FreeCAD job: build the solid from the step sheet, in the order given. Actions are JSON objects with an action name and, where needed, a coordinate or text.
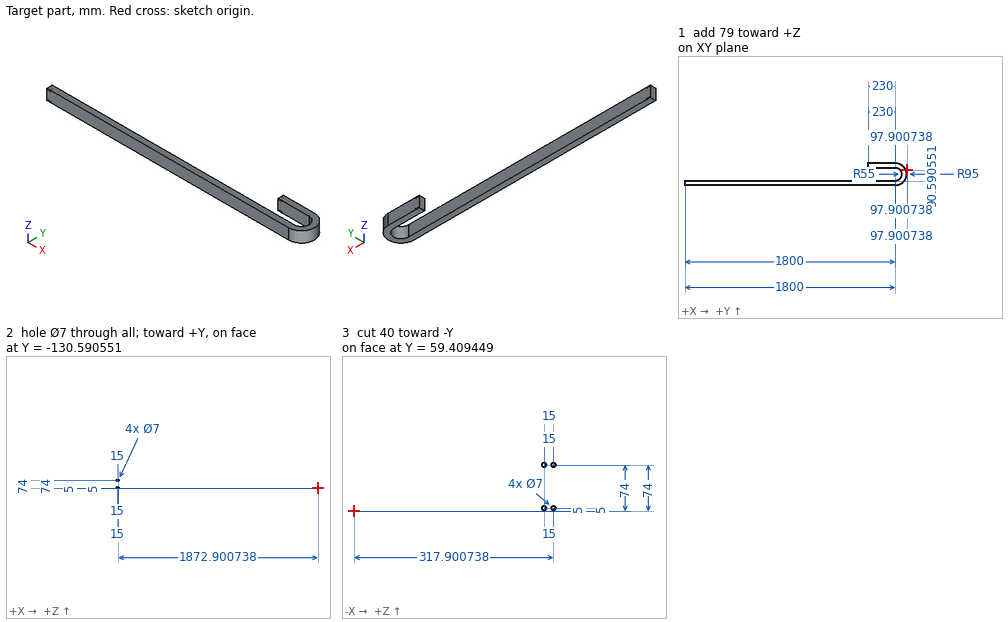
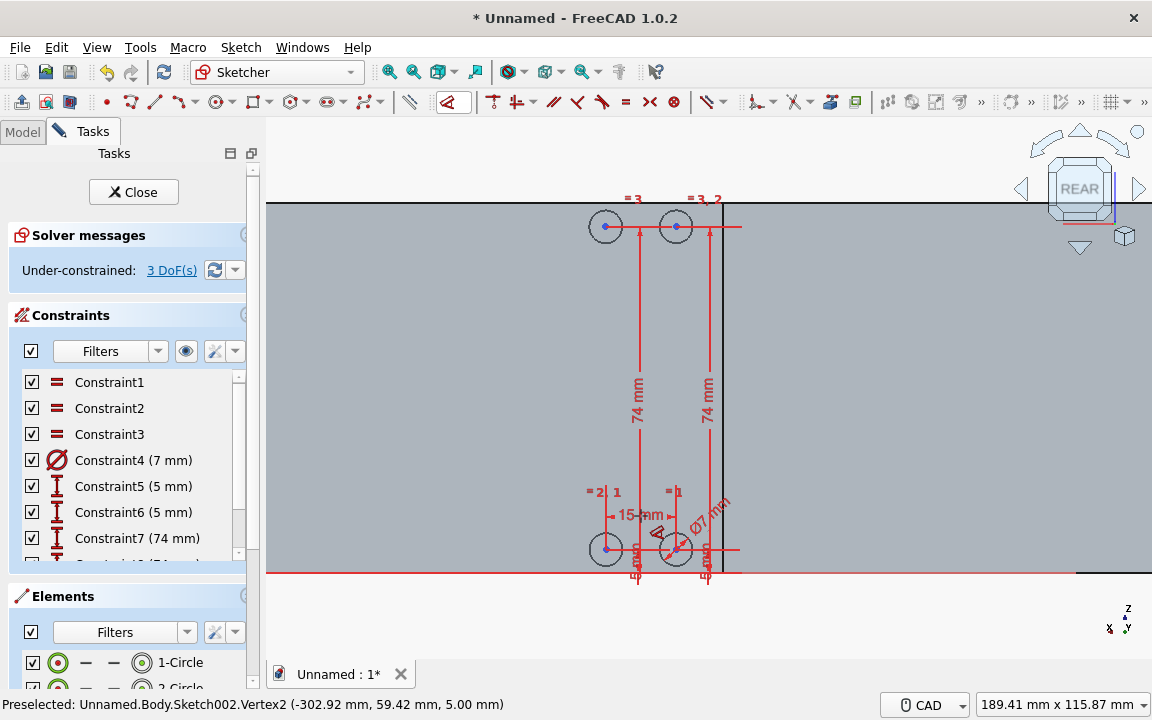
{"action": "left_click", "coordinate": [606, 550]}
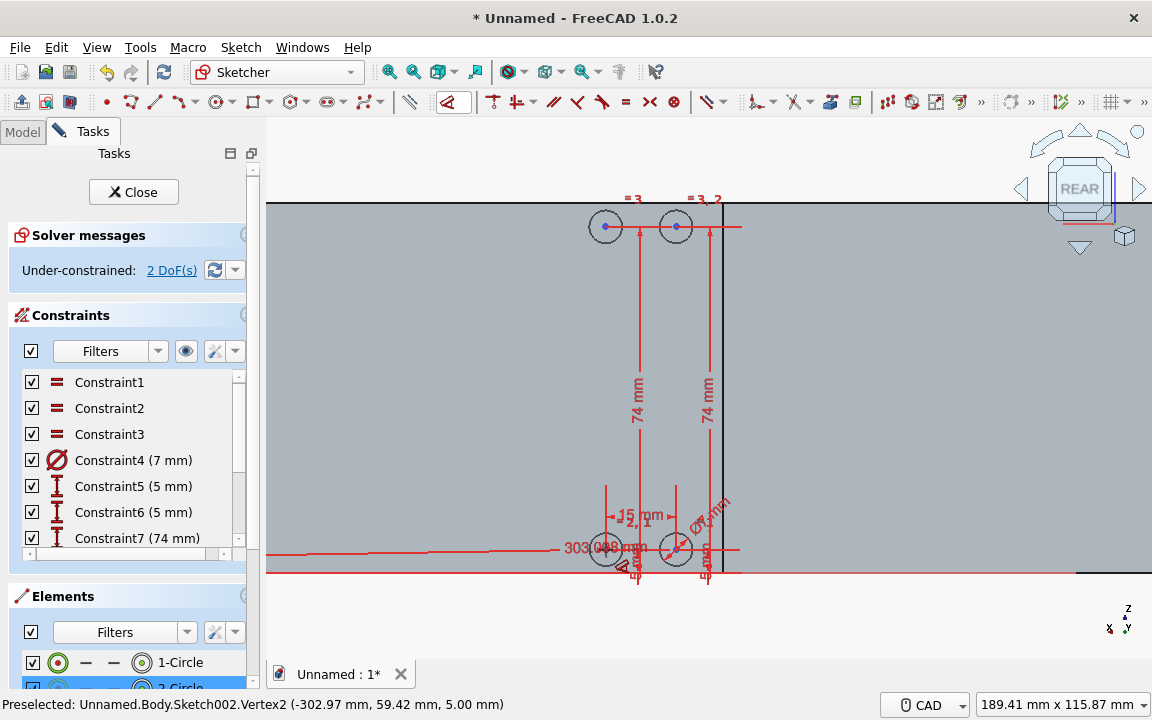
{"action": "left_click", "coordinate": [676, 227]}
{"action": "left_click", "coordinate": [641, 193]}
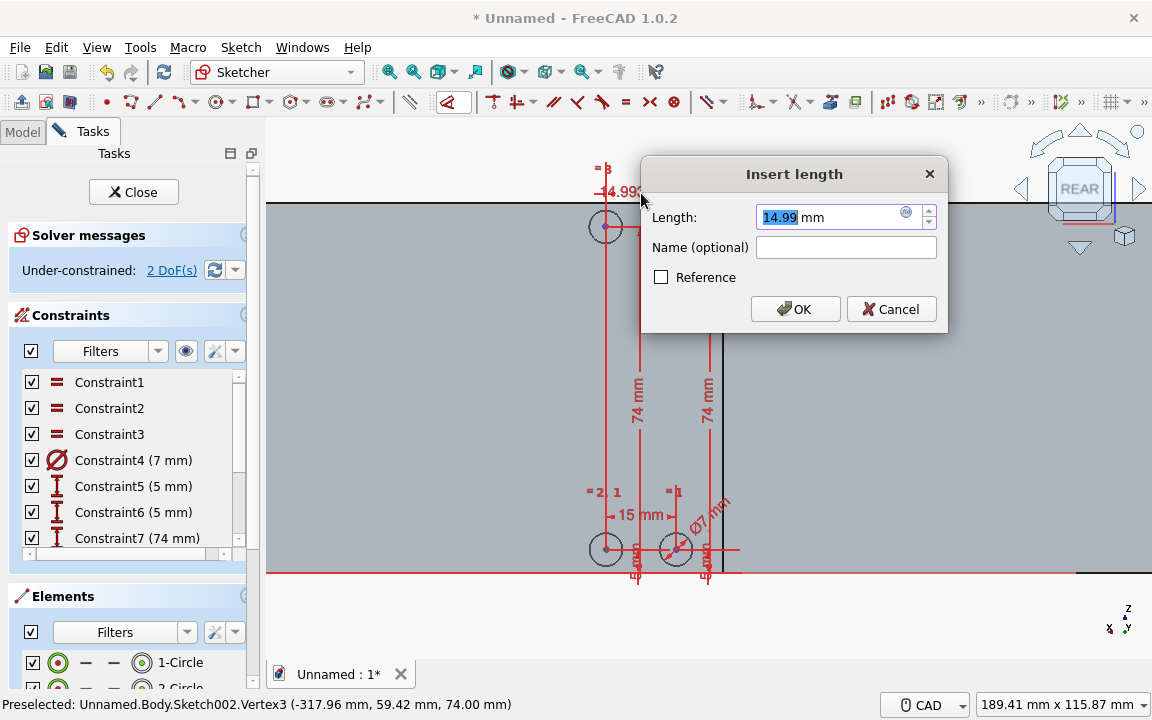
{"action": "type", "text": "15"}
{"action": "key", "text": "Return"}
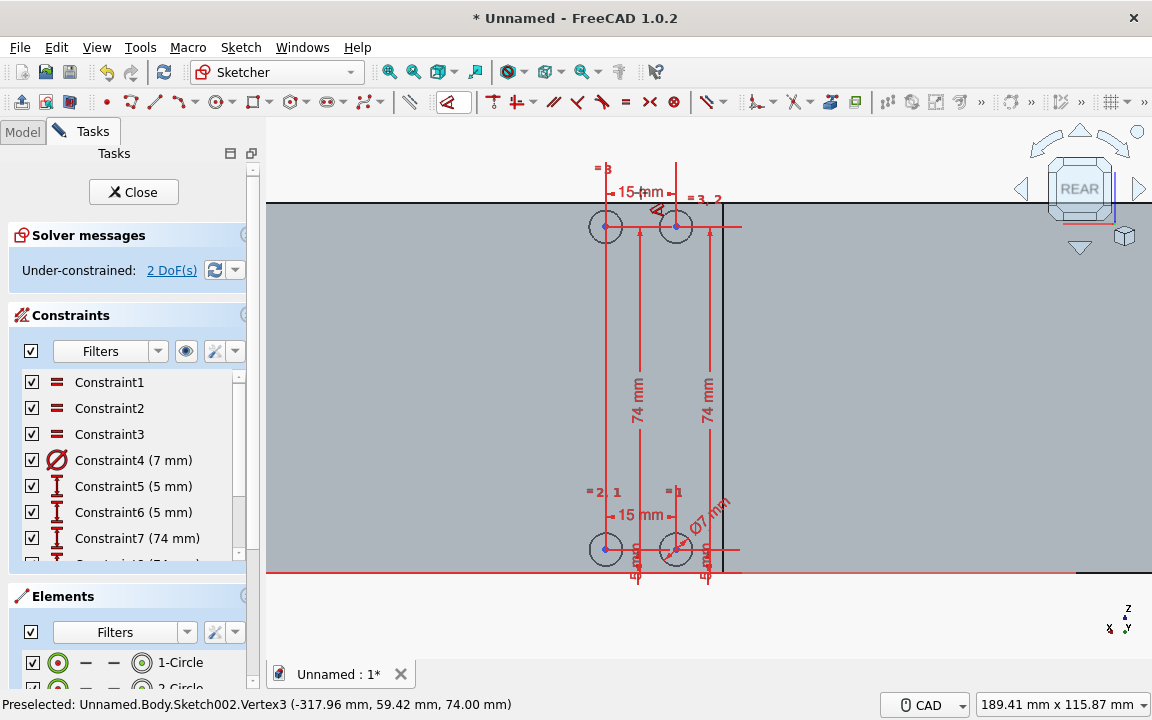
{"action": "left_click", "coordinate": [676, 227]}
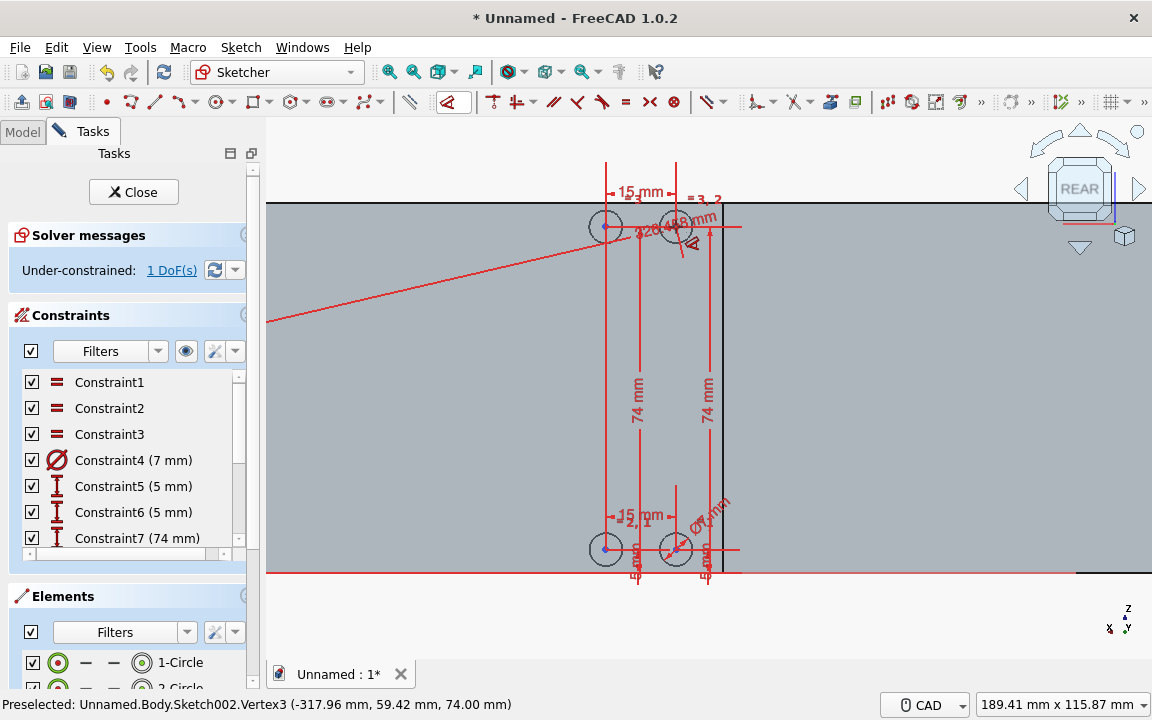
{"action": "left_click", "coordinate": [606, 227]}
{"action": "left_click", "coordinate": [641, 261]}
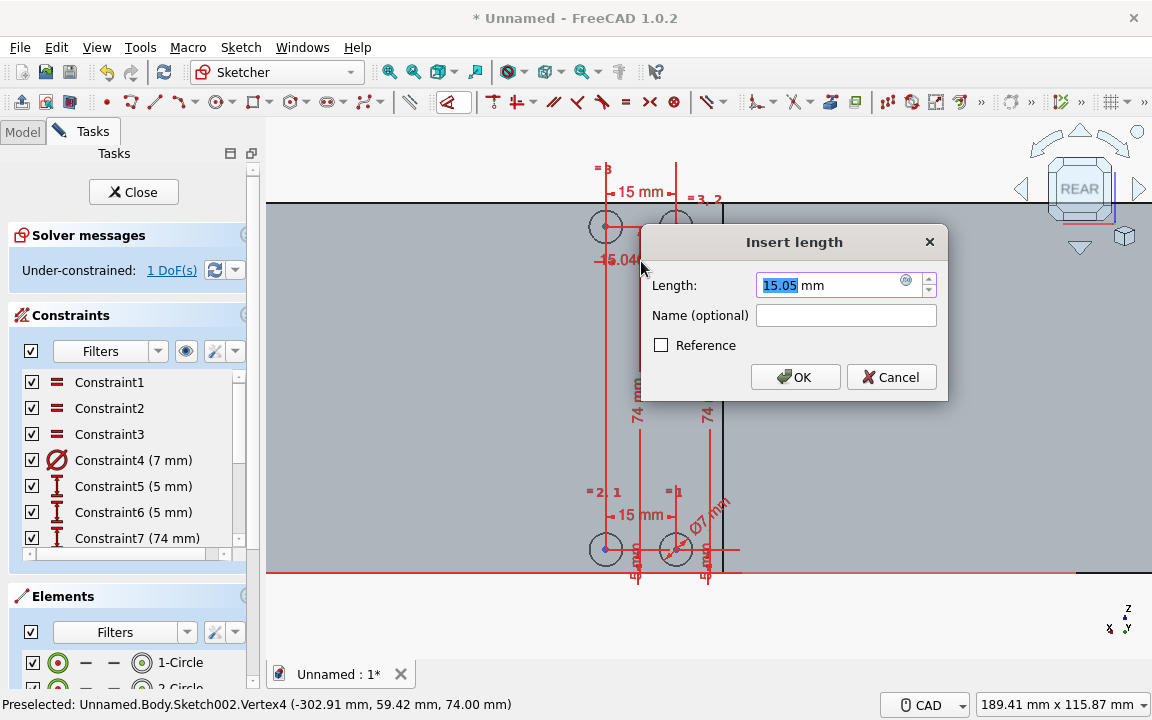
{"action": "type", "text": "15"}
{"action": "key", "text": "Return"}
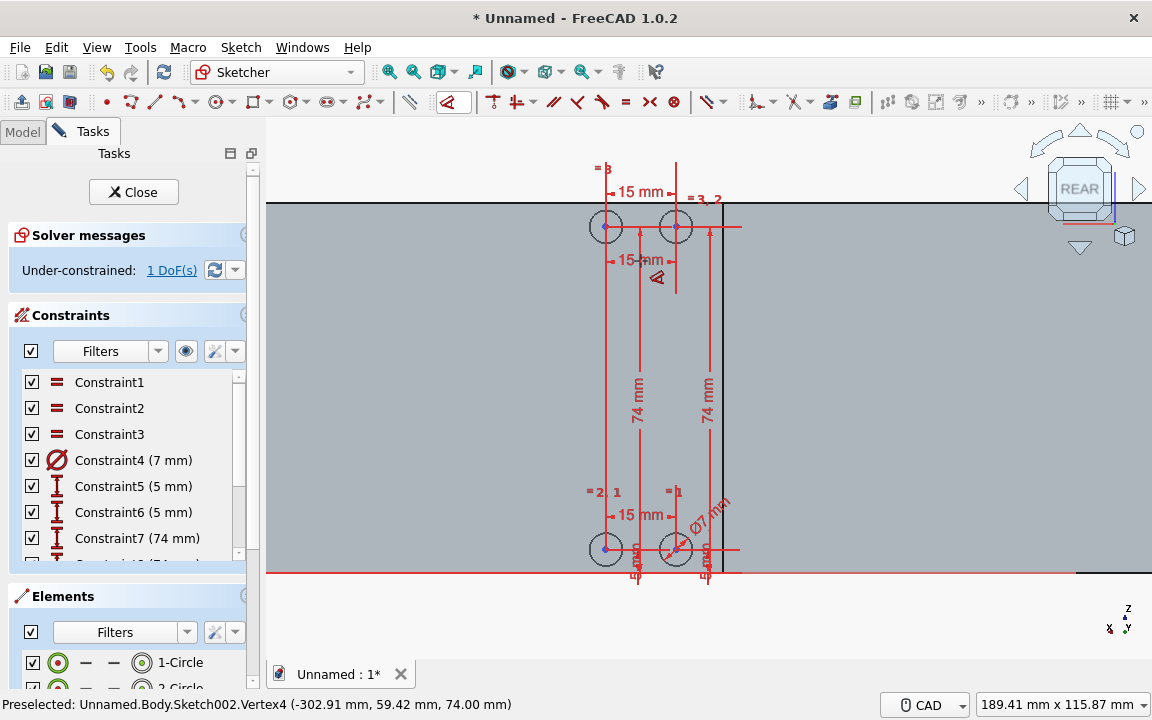
{"action": "left_click", "coordinate": [676, 550]}
{"action": "left_click", "coordinate": [485, 607]}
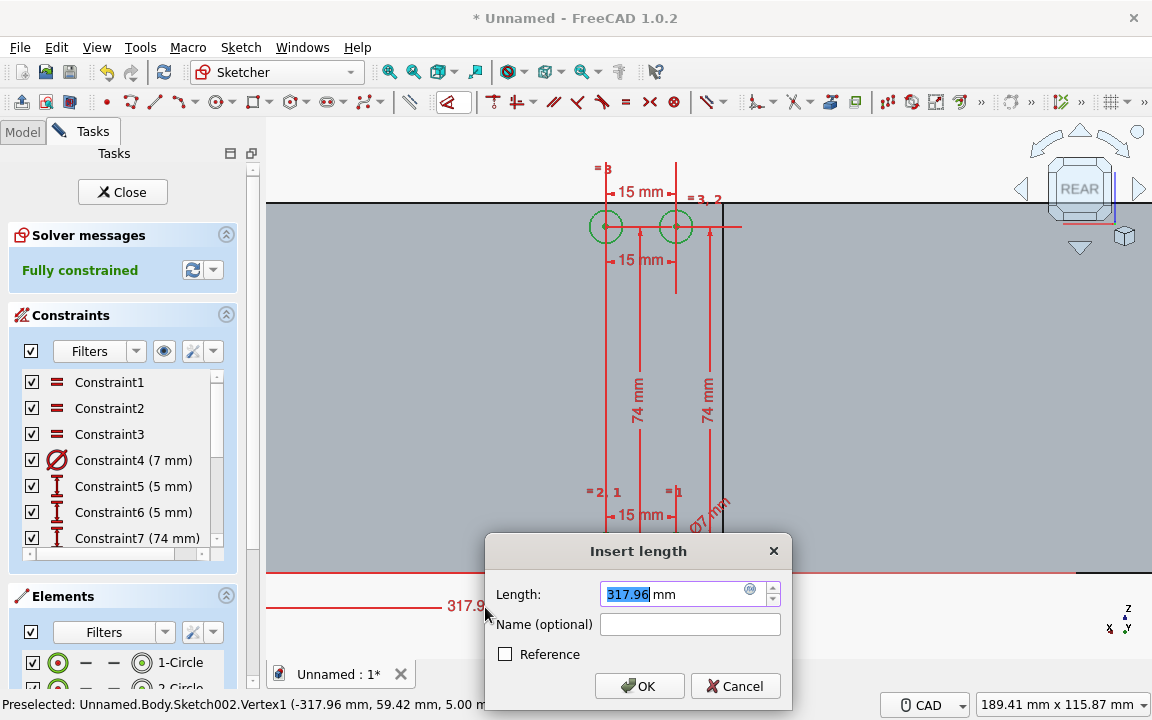
{"action": "type", "text": "317.900738"}
{"action": "key", "text": "Return"}
{"action": "key", "text": "Escape"}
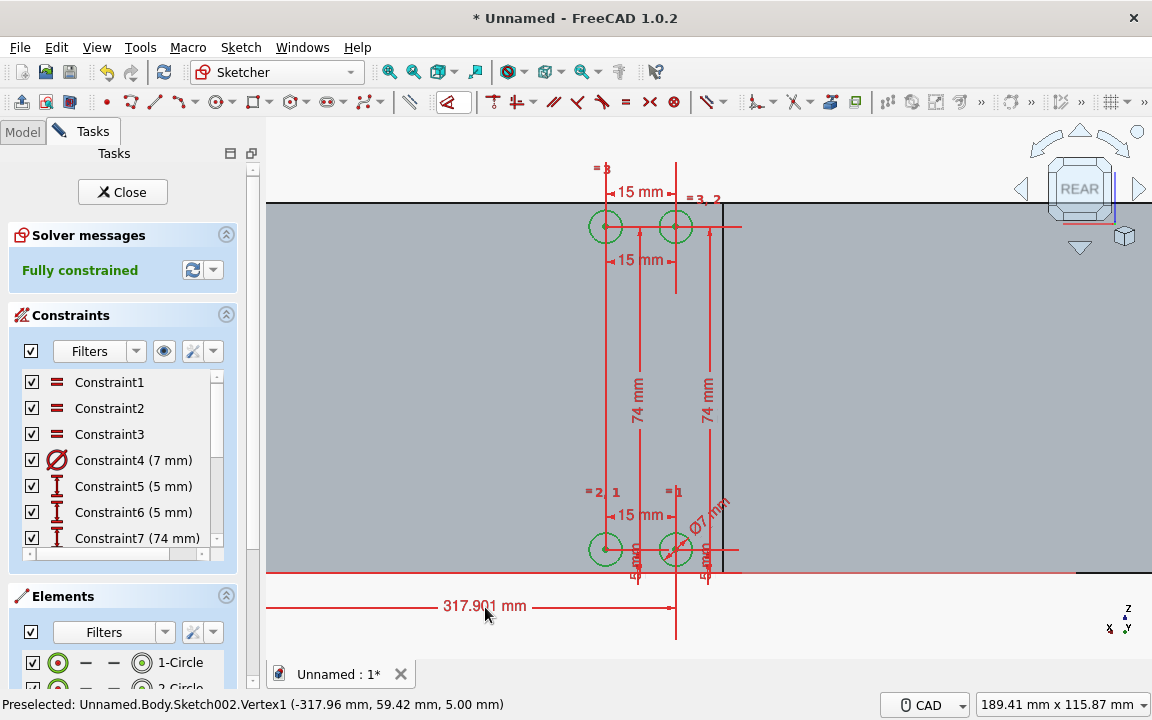
{"action": "left_click", "coordinate": [123, 192]}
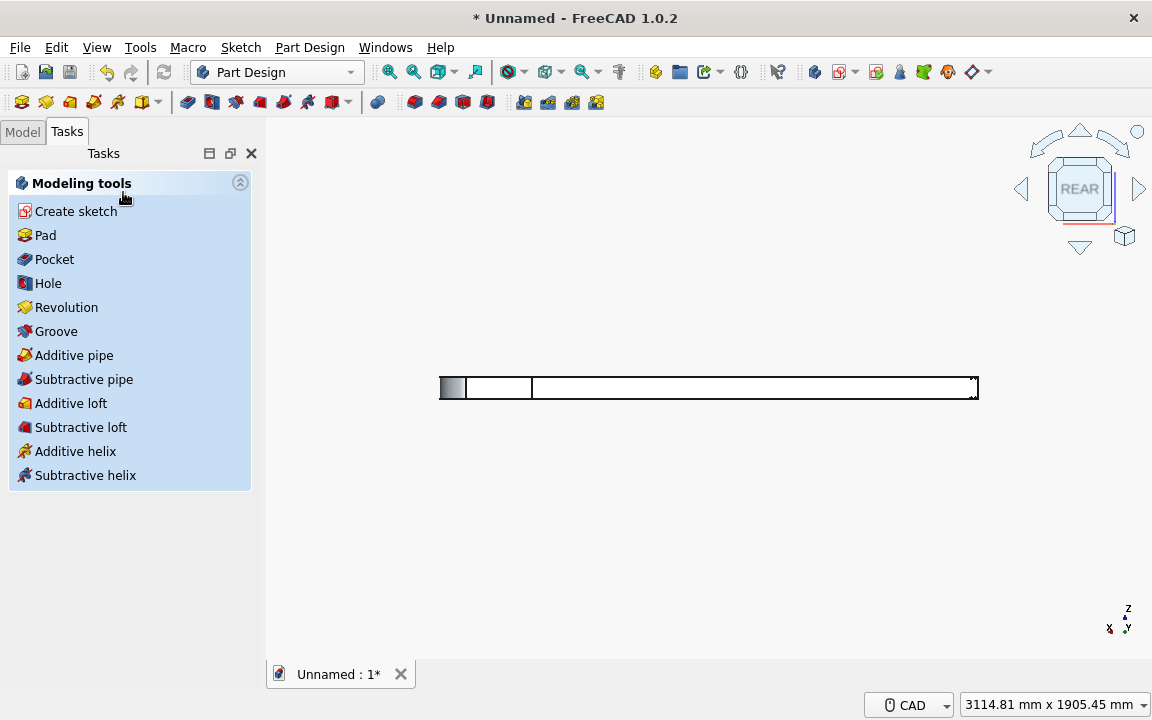
{"action": "left_click", "coordinate": [188, 102]}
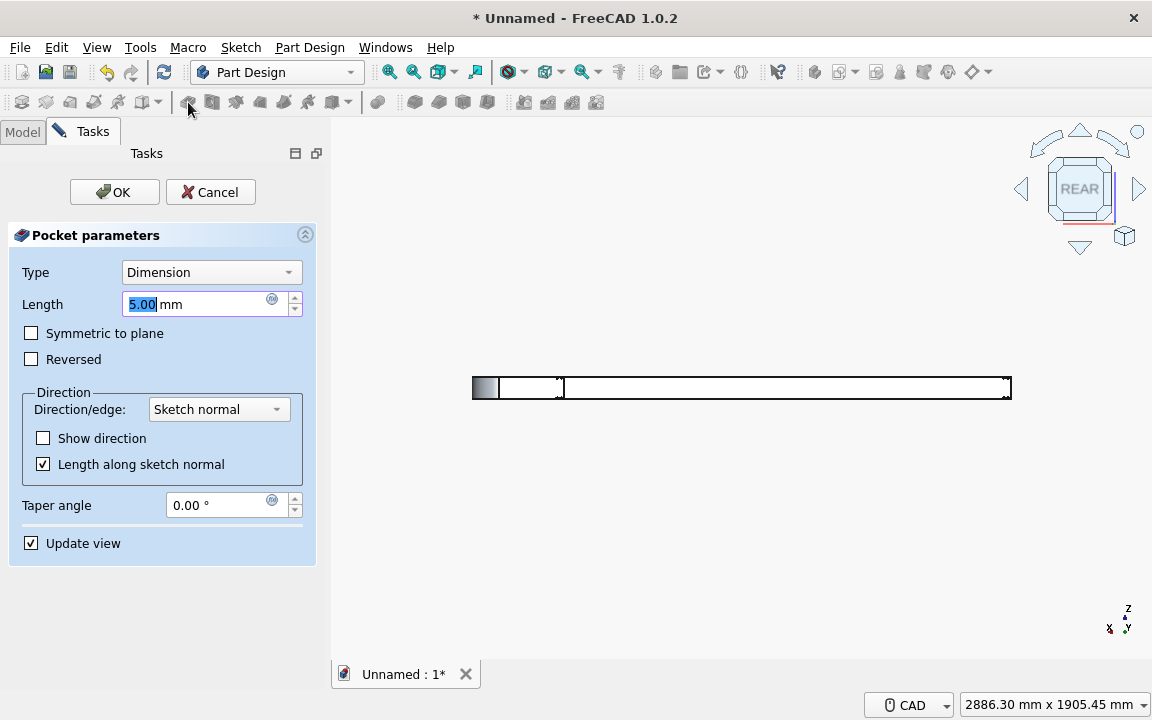
{"action": "type", "text": "40"}
{"action": "key", "text": "Tab"}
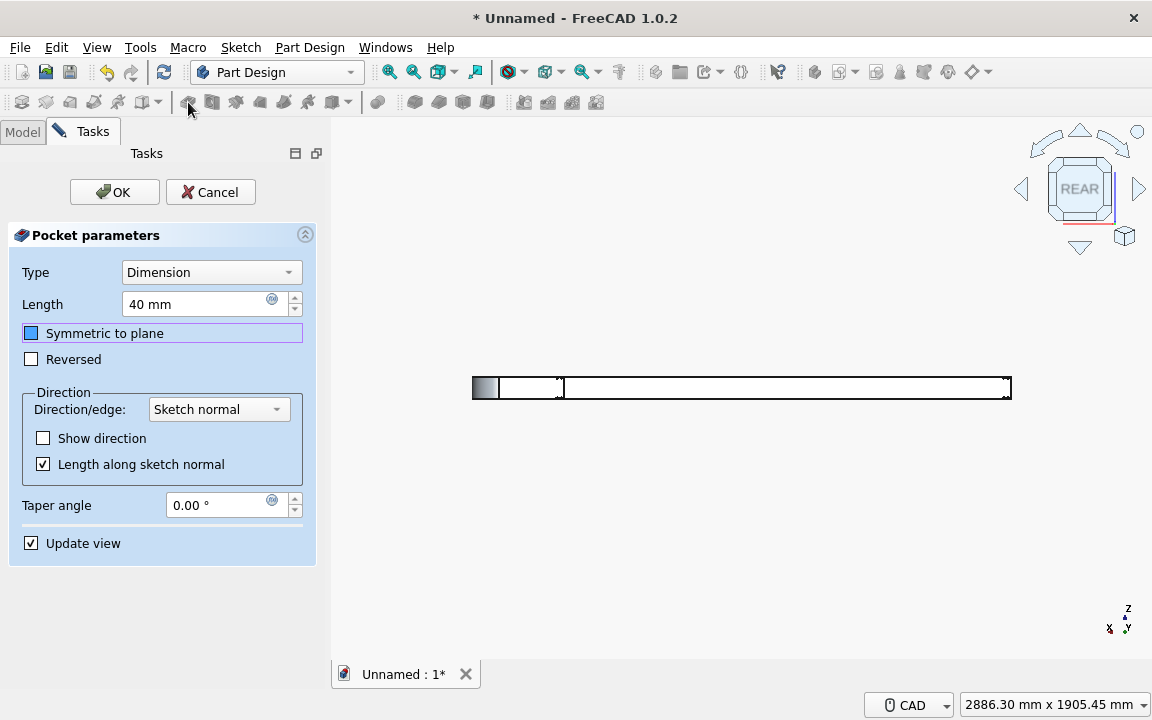
{"action": "left_click", "coordinate": [115, 192]}